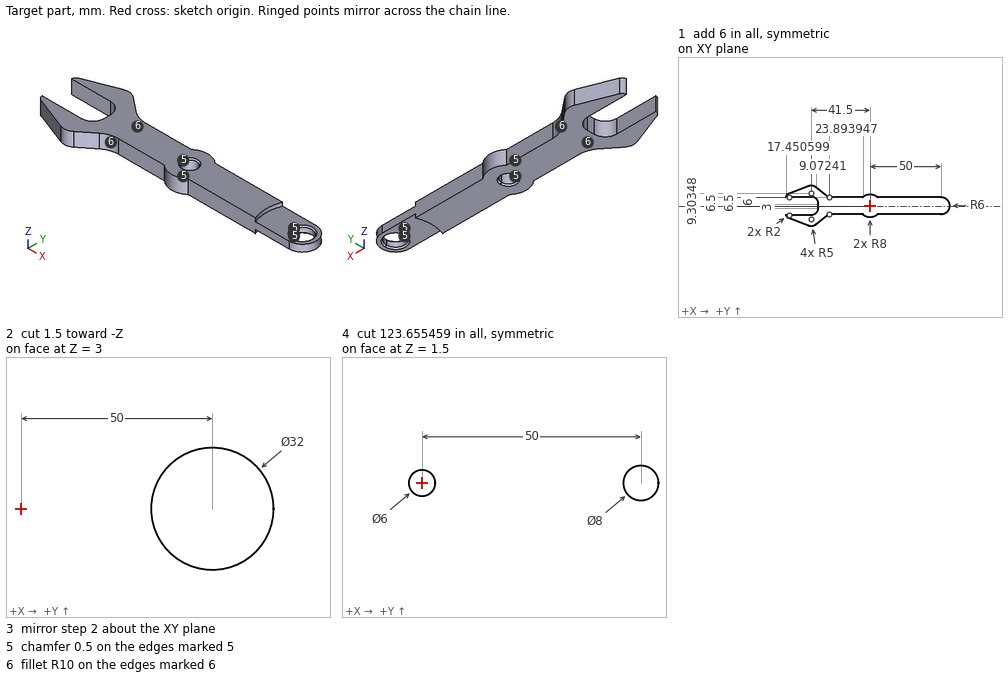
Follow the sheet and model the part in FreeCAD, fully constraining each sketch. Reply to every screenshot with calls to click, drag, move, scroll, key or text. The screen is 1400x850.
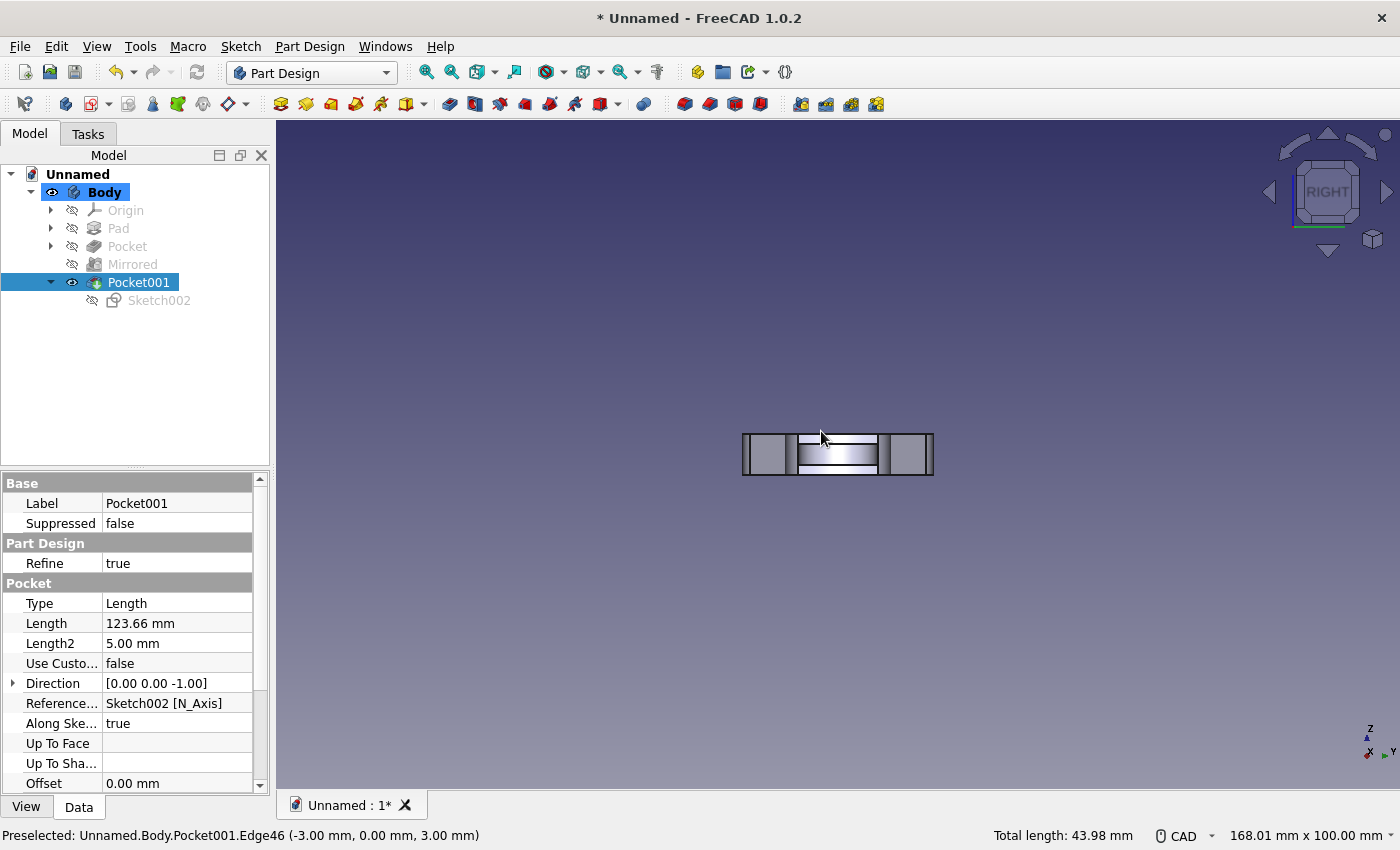
click(427, 72)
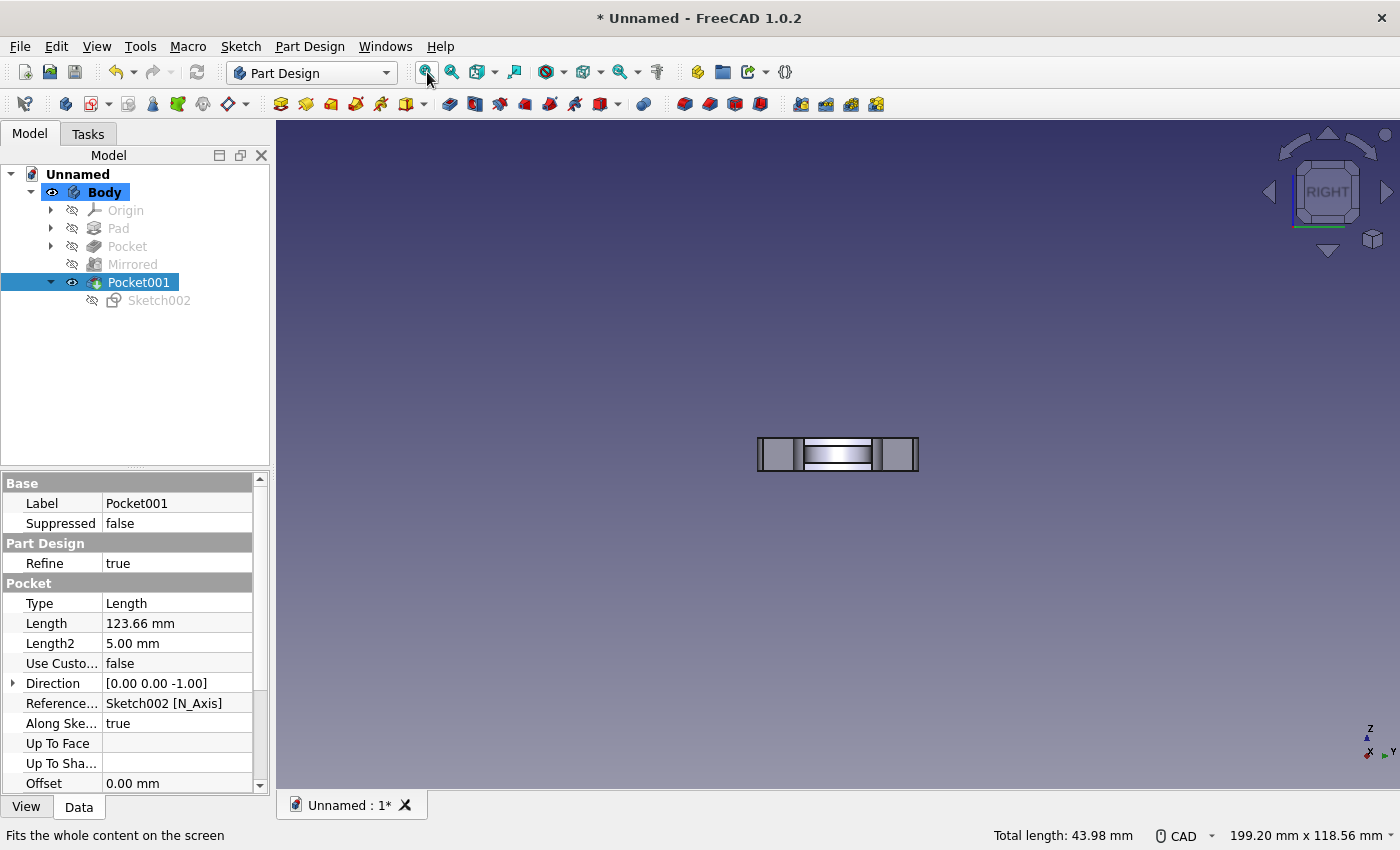
key(5)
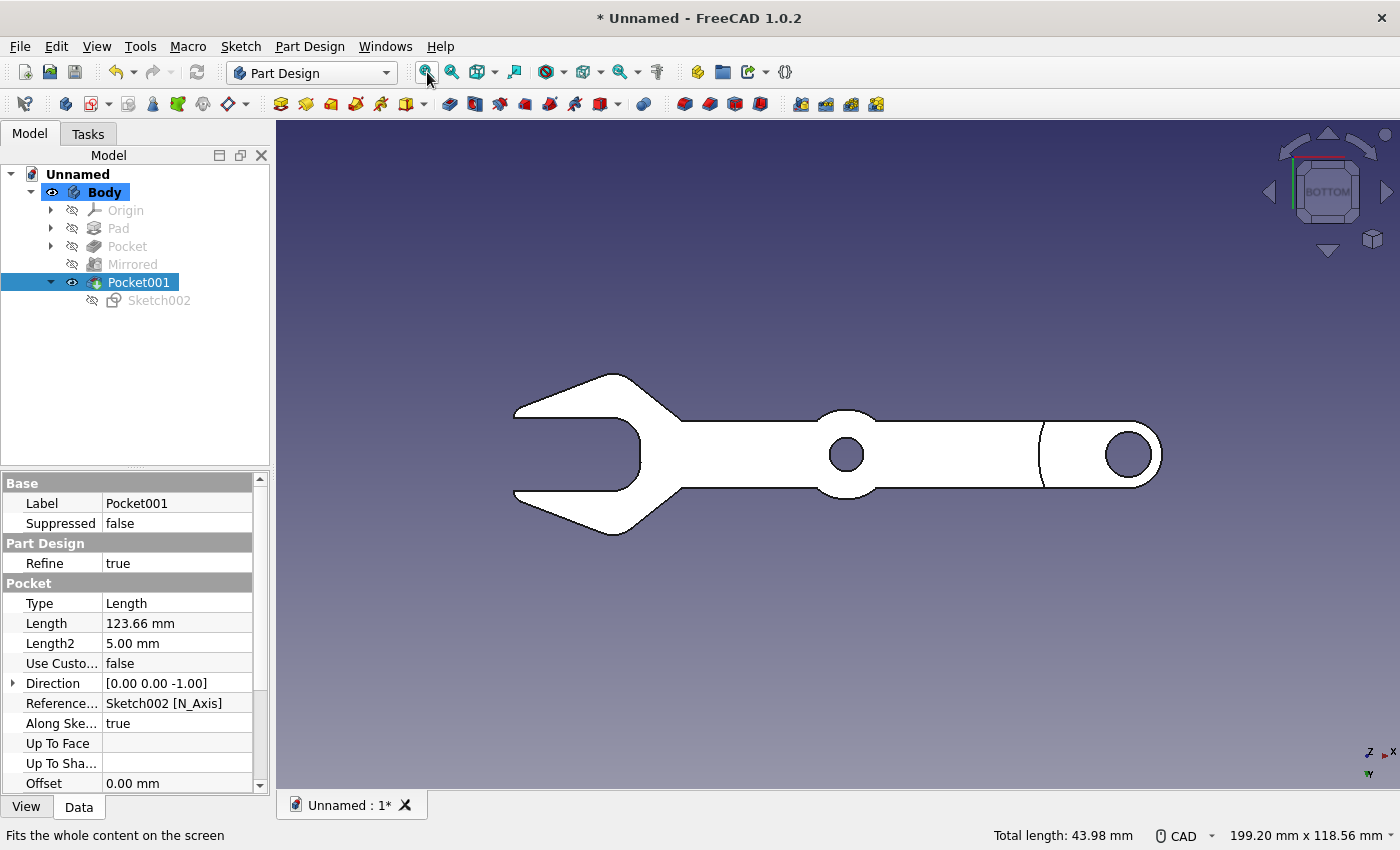
click(1106, 453, ctrl)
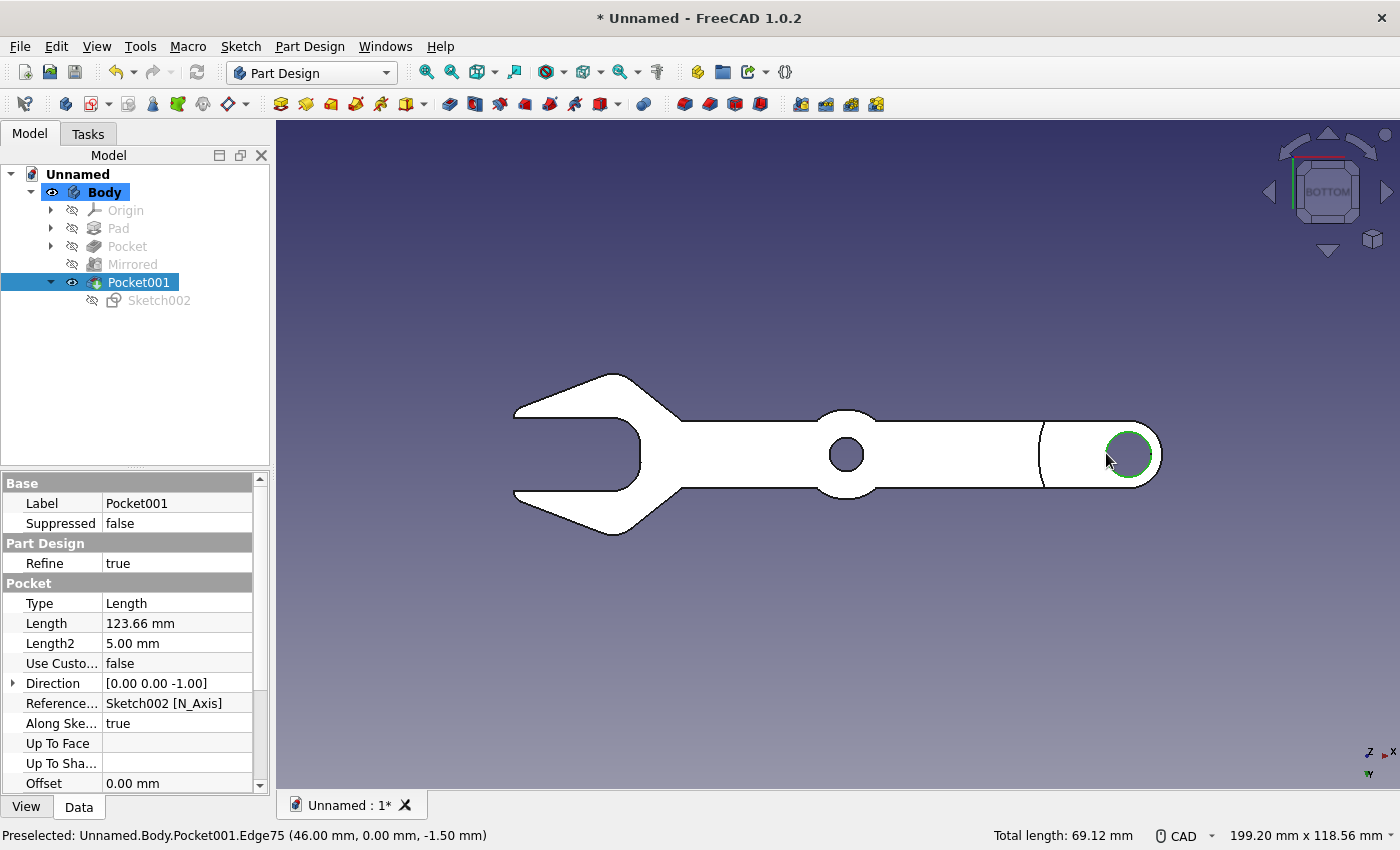
click(830, 453, ctrl)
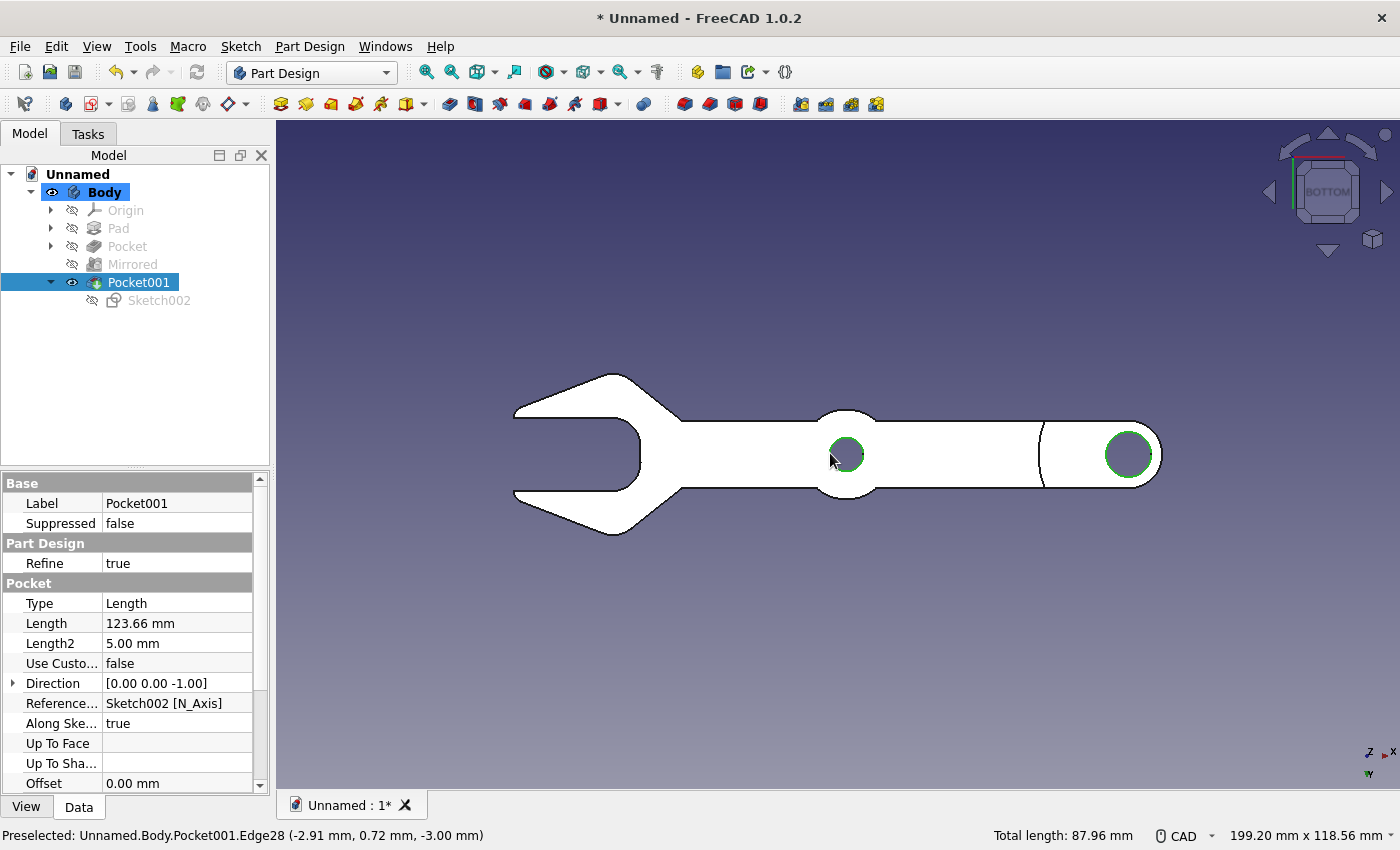
click(710, 104)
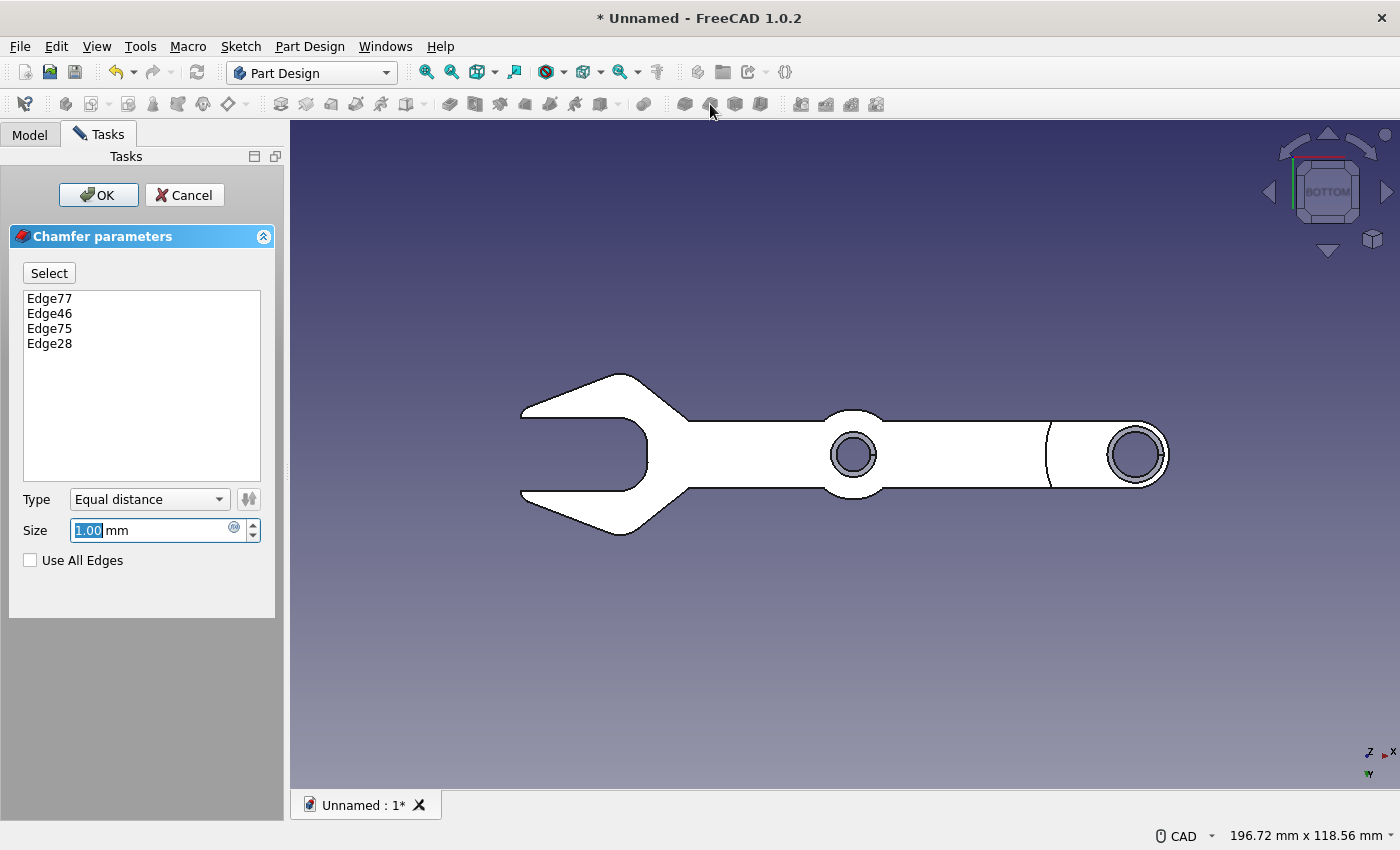
text(0.5)
key(Tab)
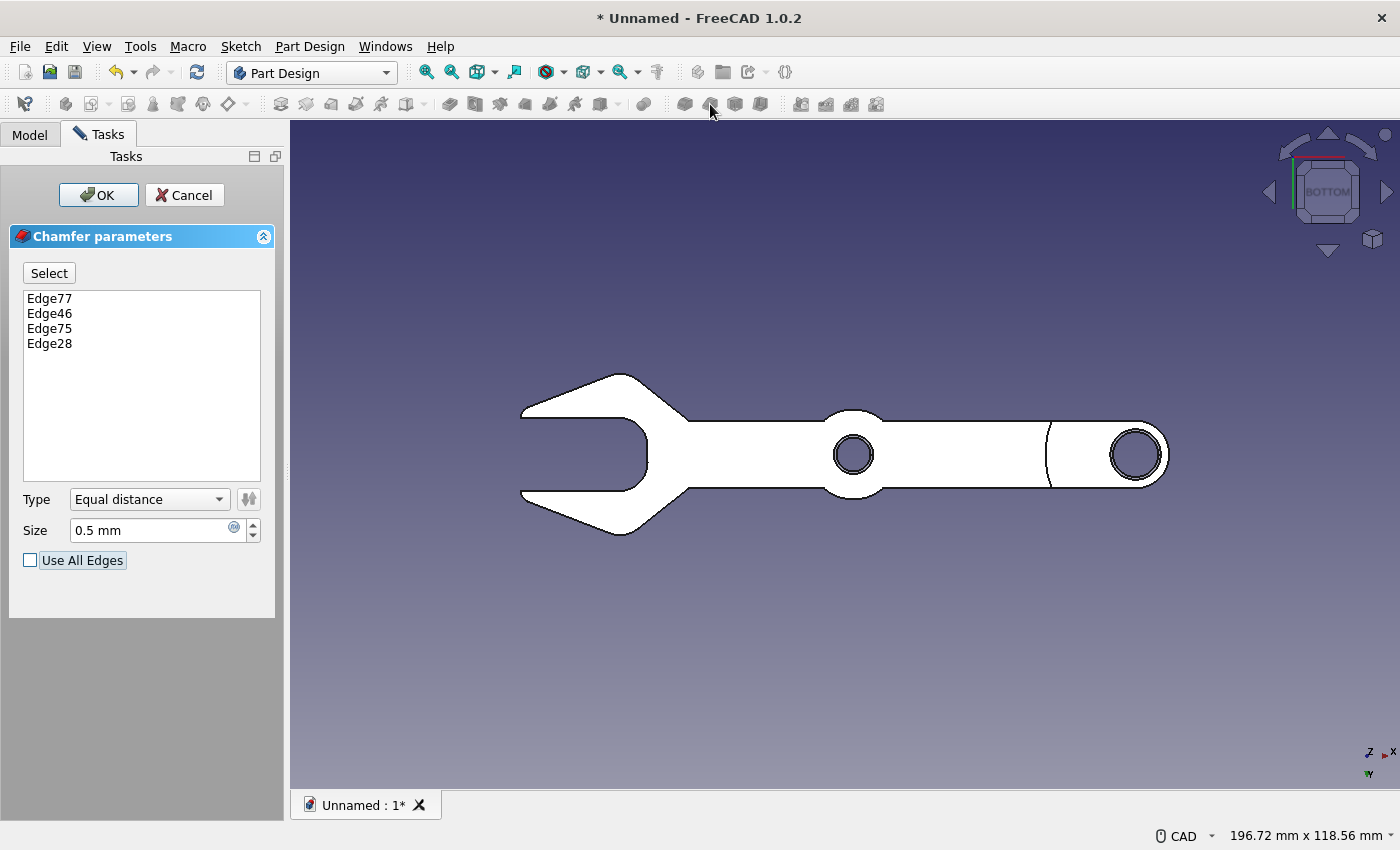
click(99, 195)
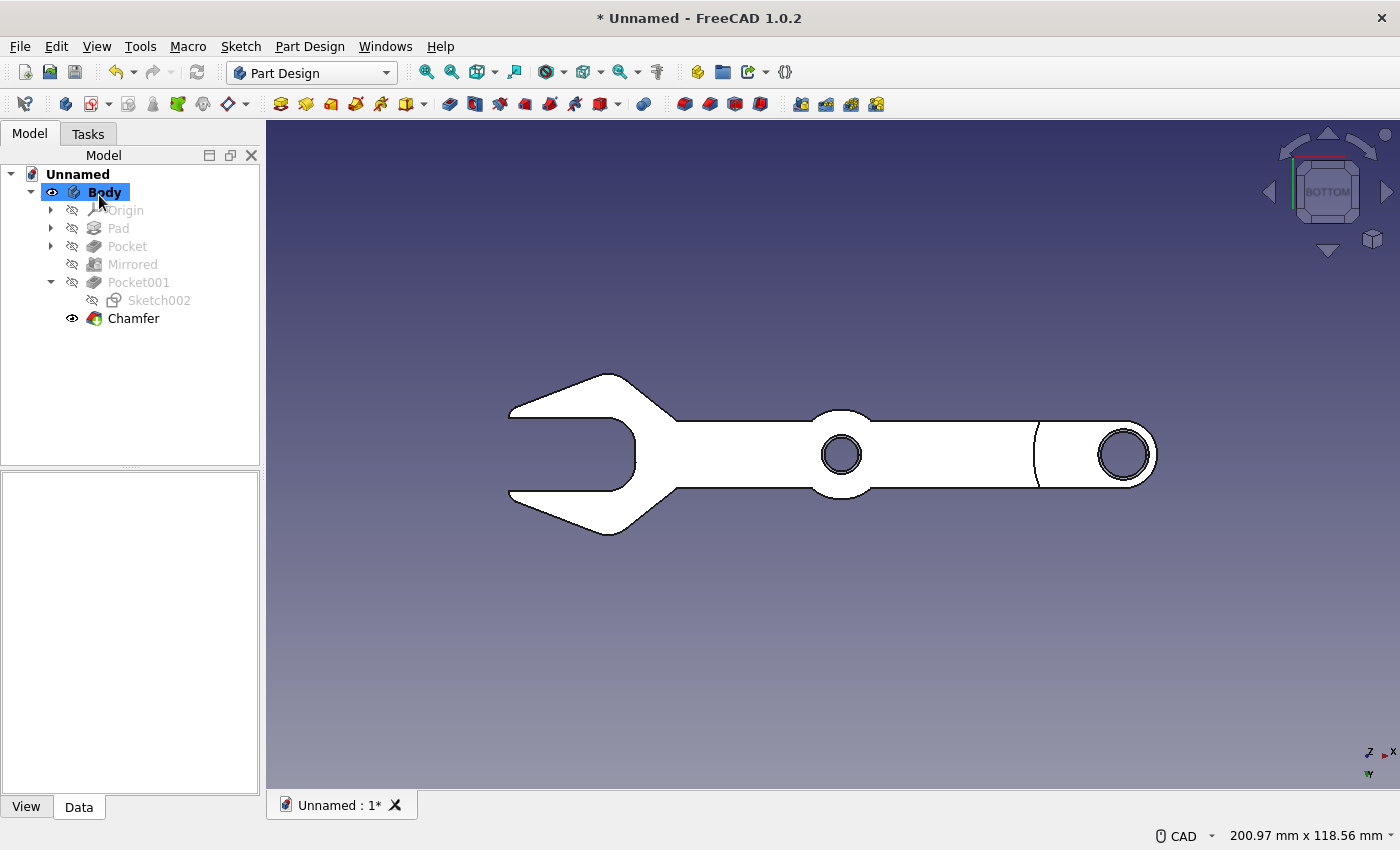
key(0)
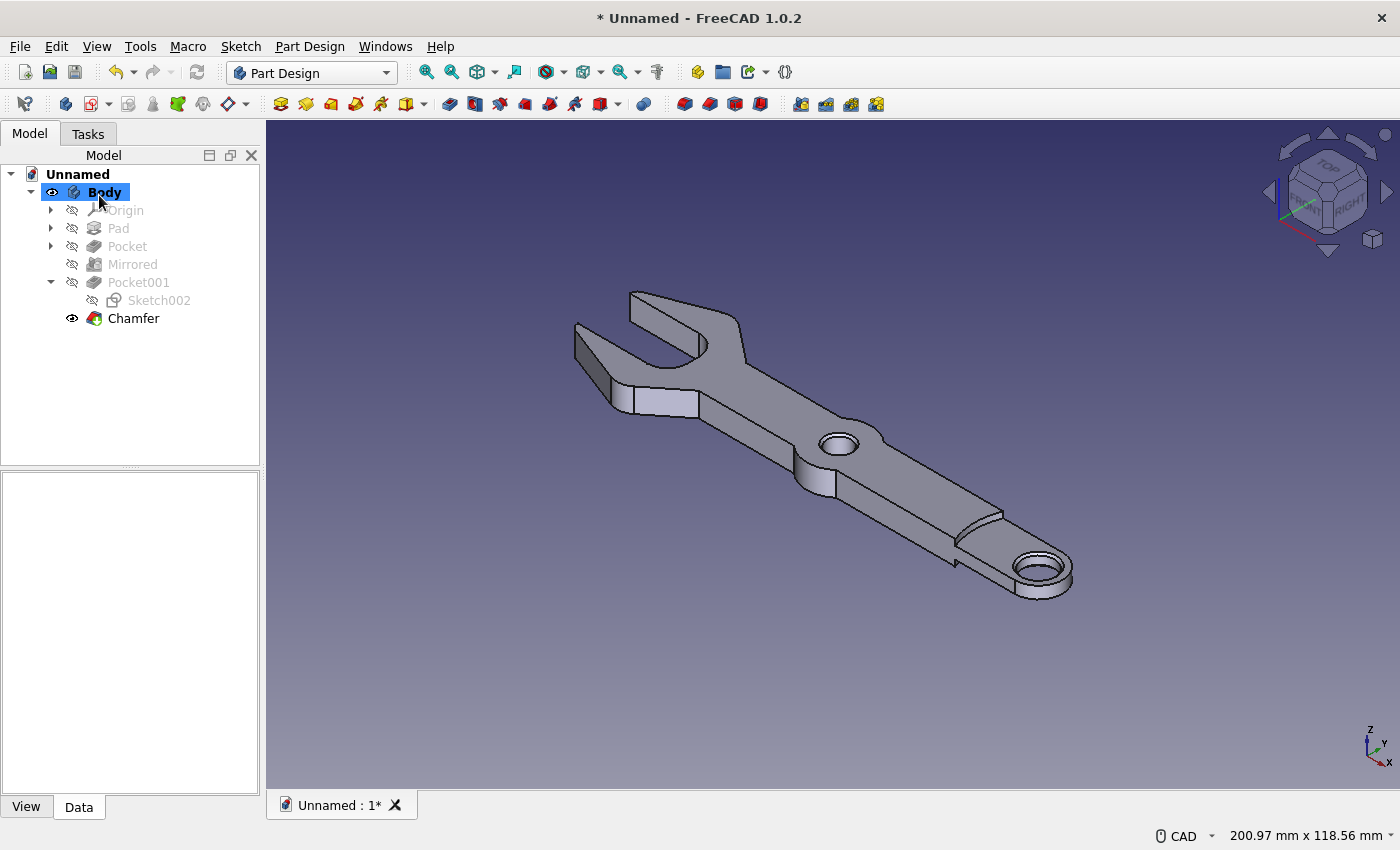
key(2)